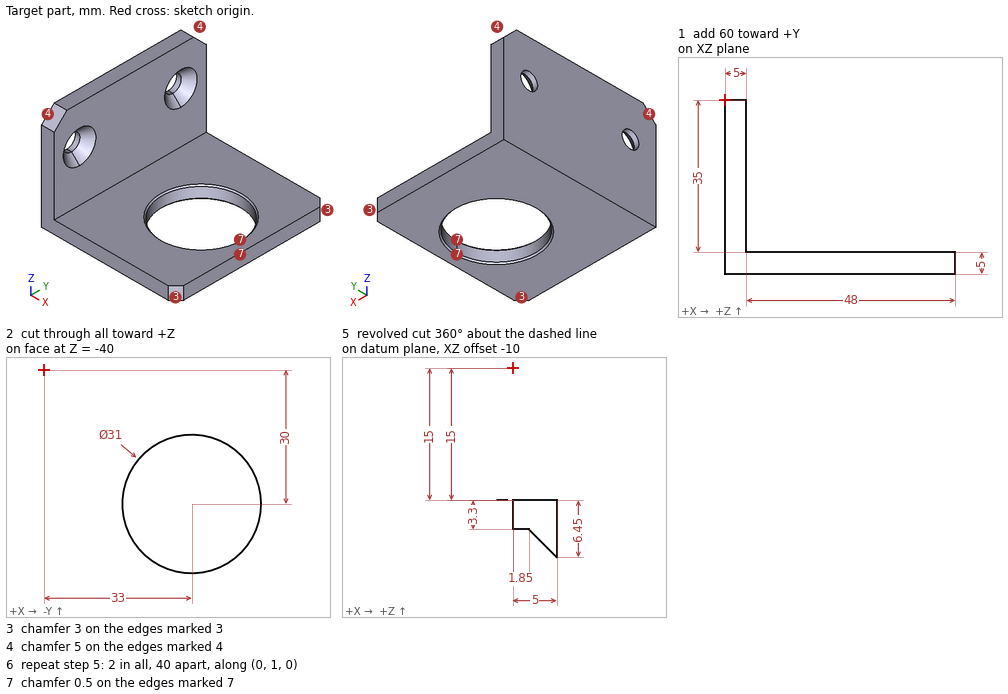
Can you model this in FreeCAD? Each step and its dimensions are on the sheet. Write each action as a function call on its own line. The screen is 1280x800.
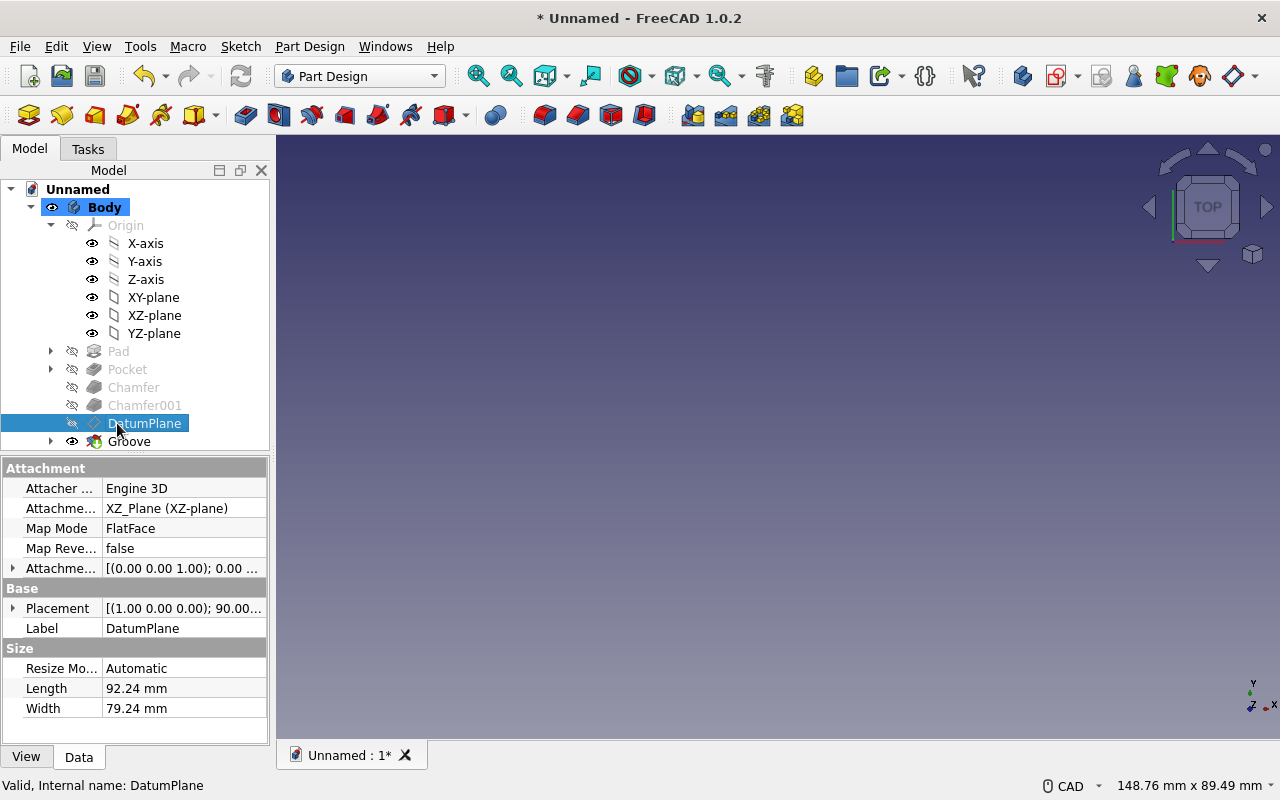
key(v)
key(f)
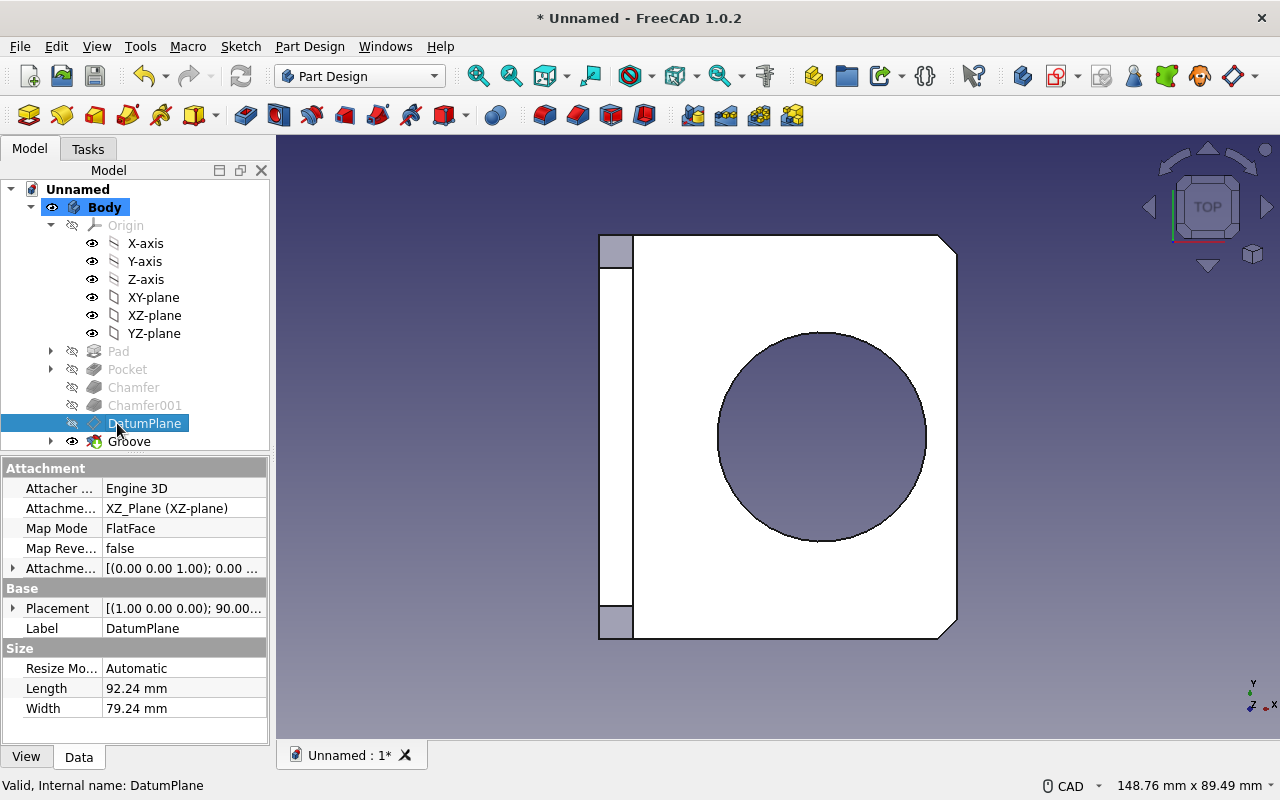
click(117, 441)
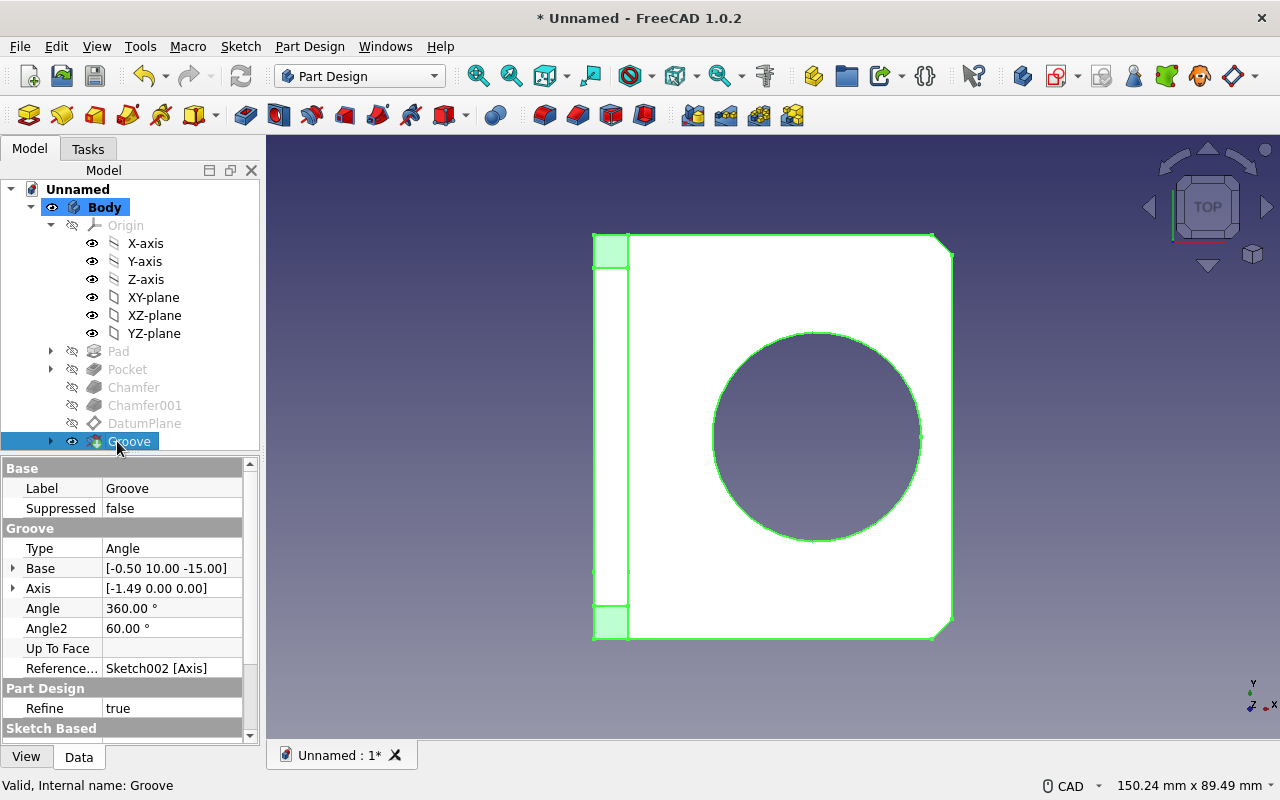
click(726, 116)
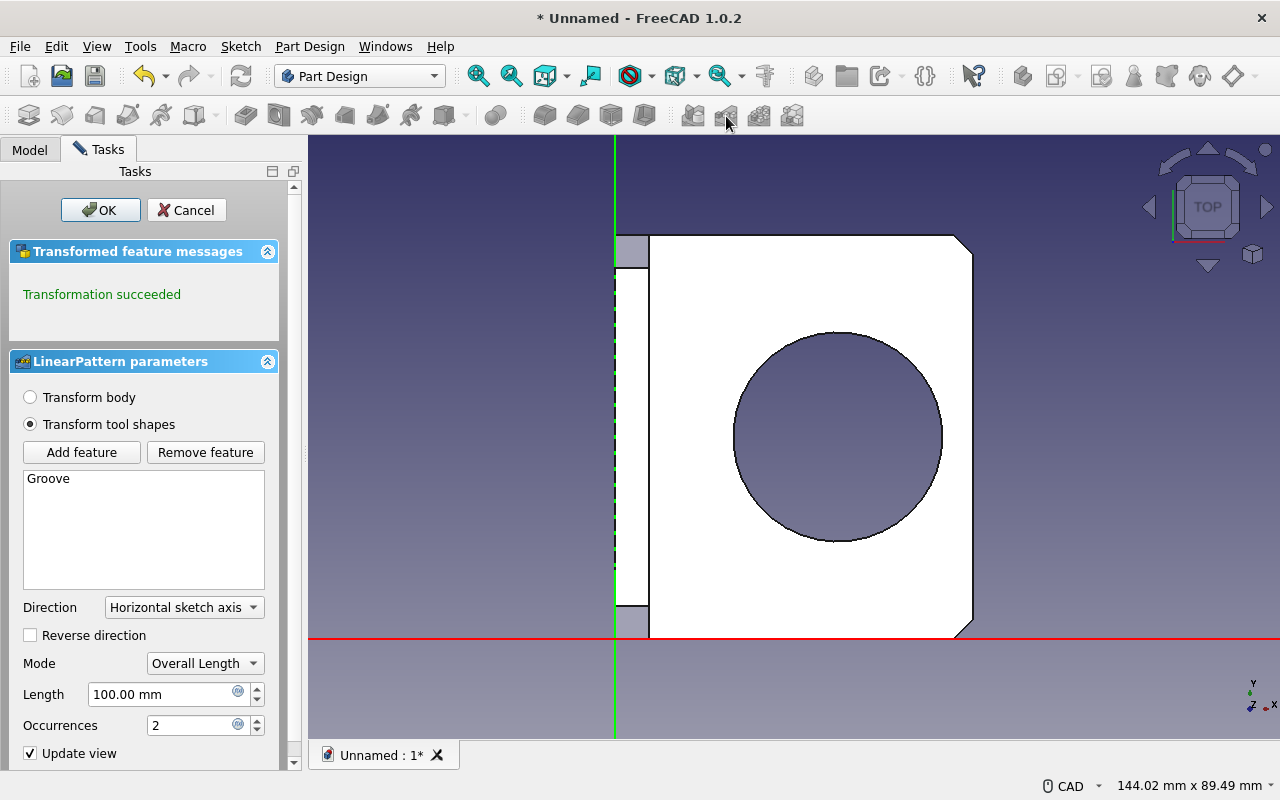
click(185, 608)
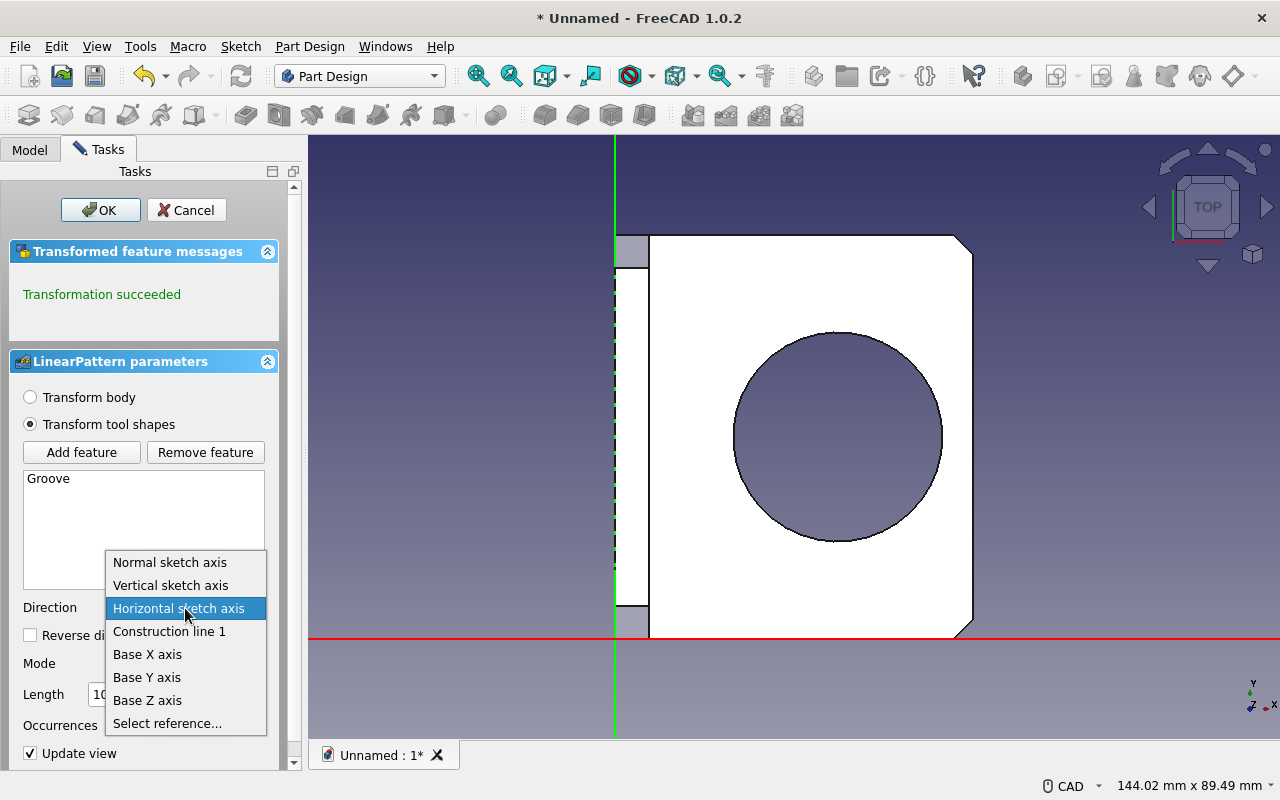
click(184, 678)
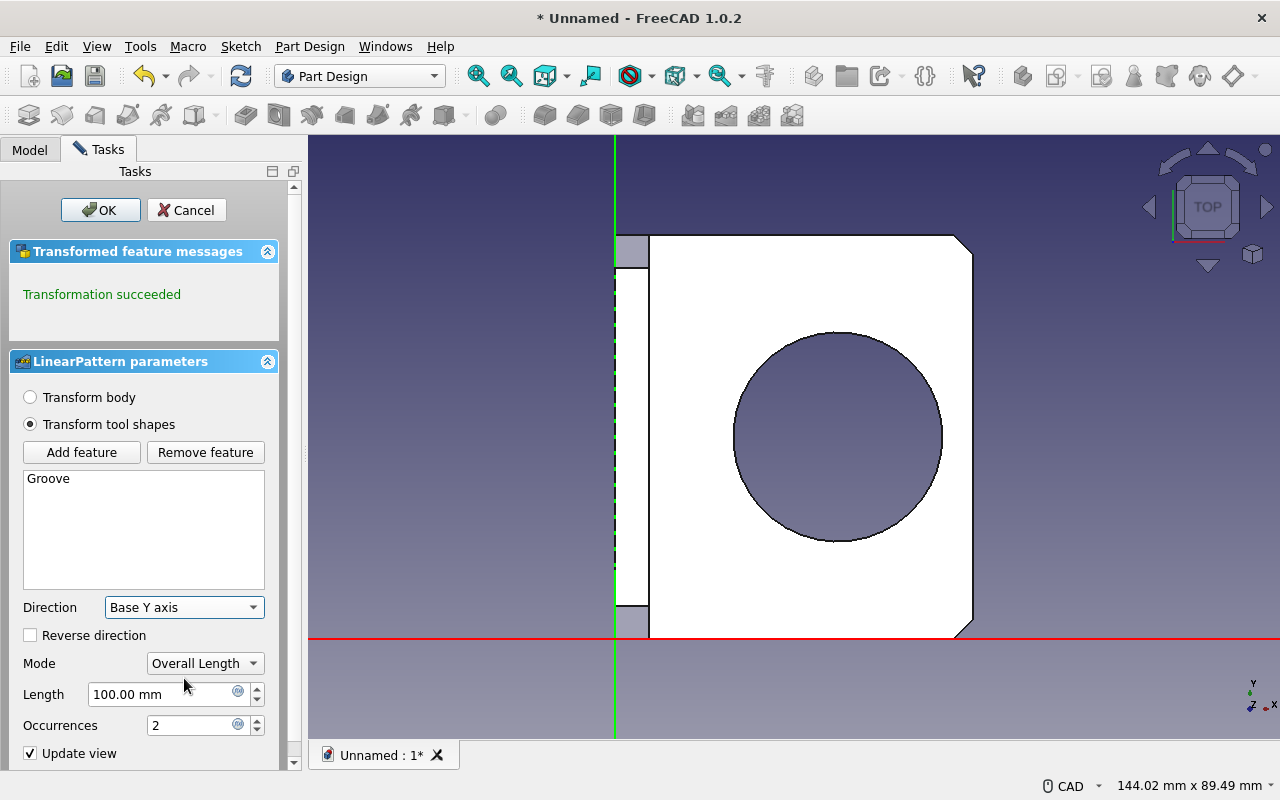
click(206, 664)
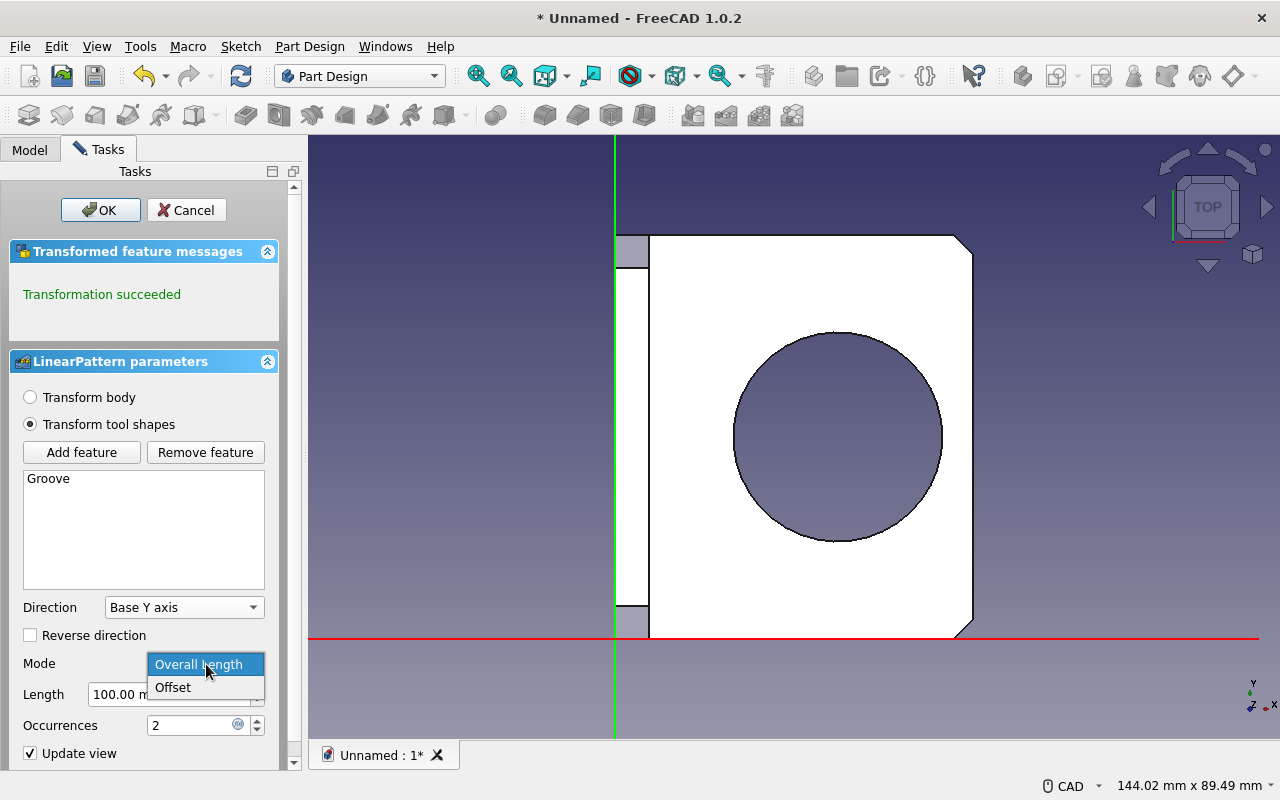
click(204, 688)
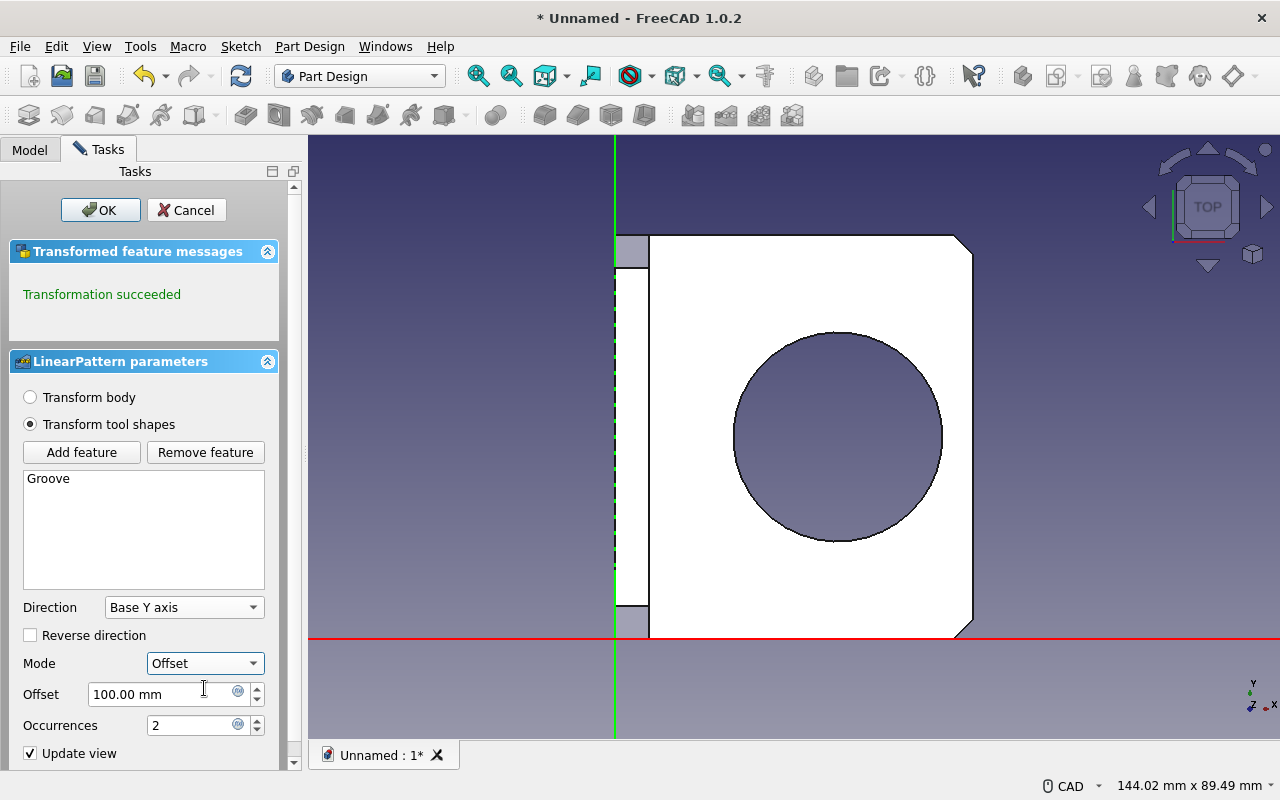
triple_click(170, 694)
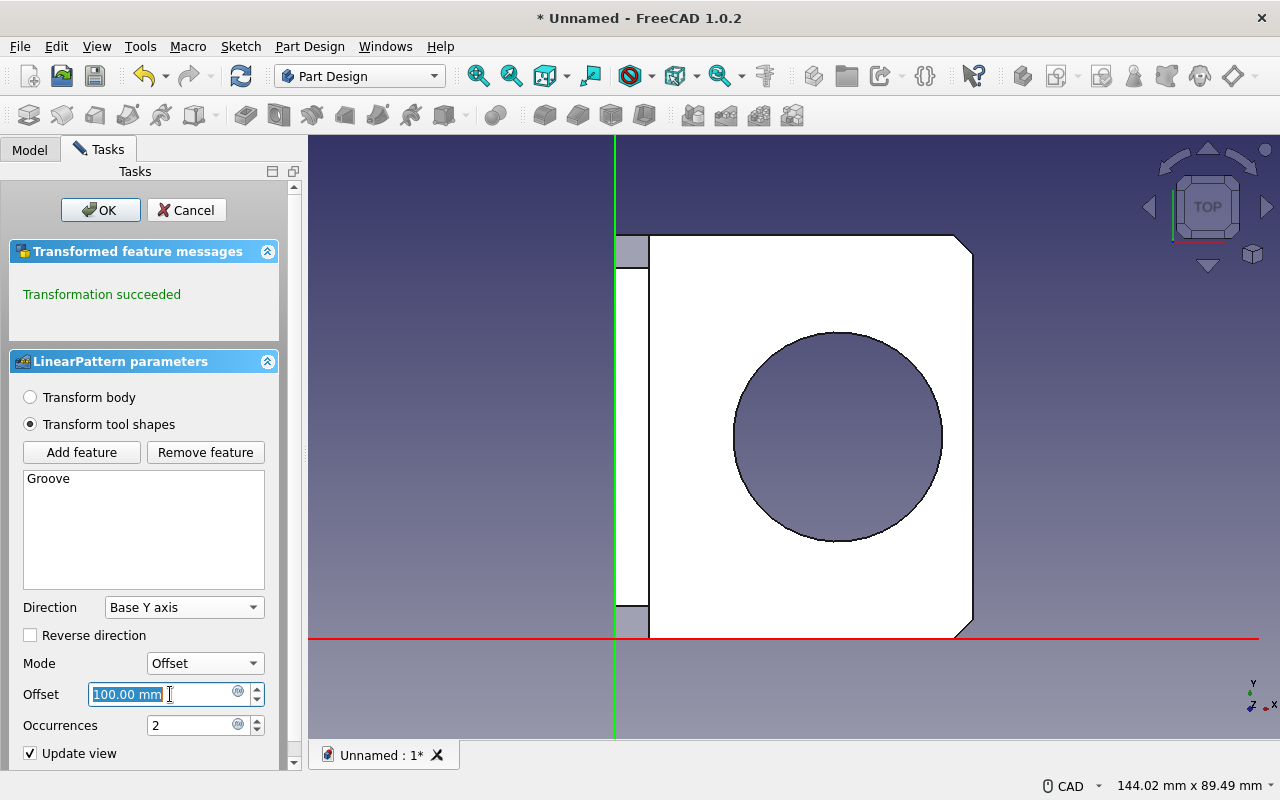
text(40)
key(Tab)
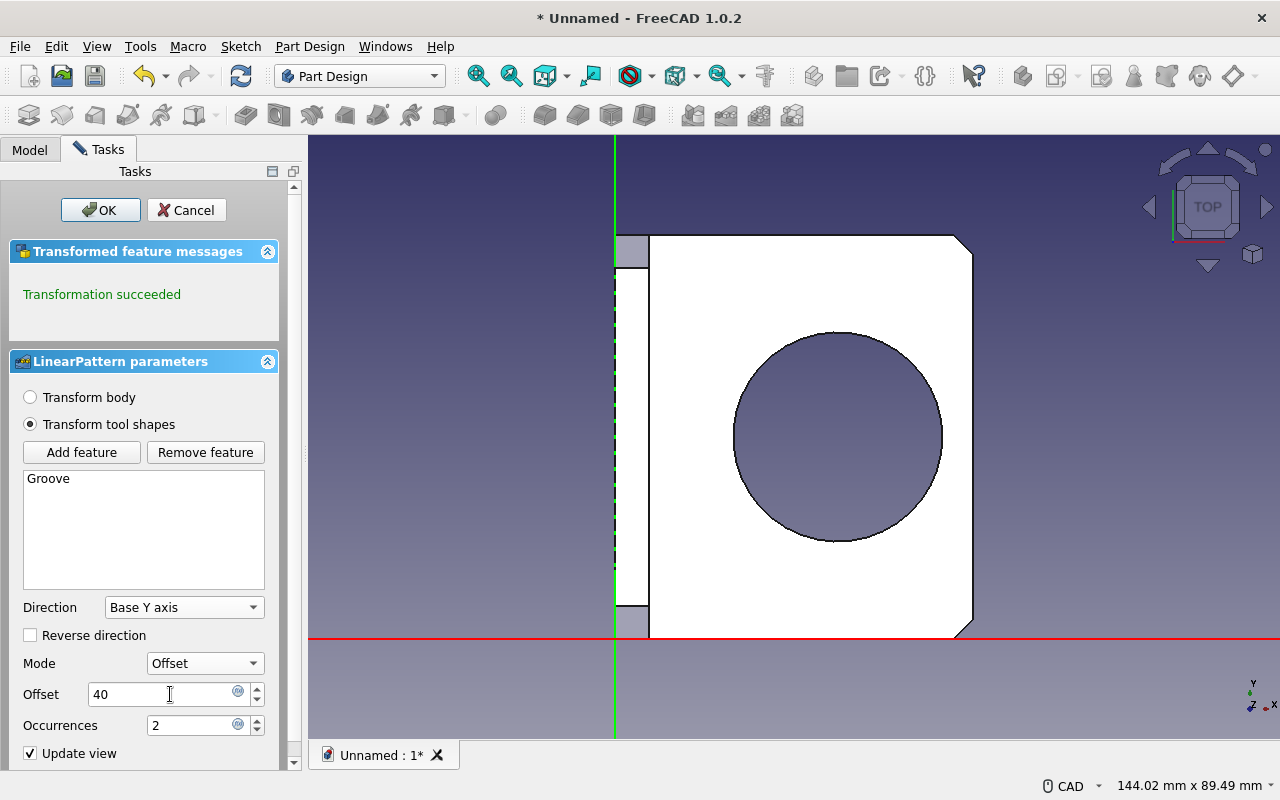
triple_click(199, 726)